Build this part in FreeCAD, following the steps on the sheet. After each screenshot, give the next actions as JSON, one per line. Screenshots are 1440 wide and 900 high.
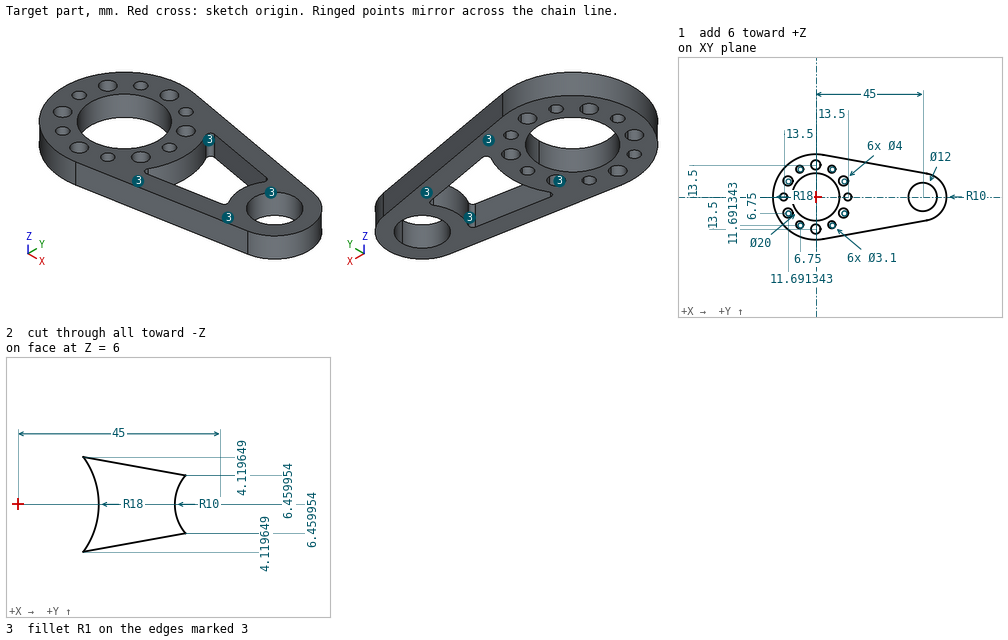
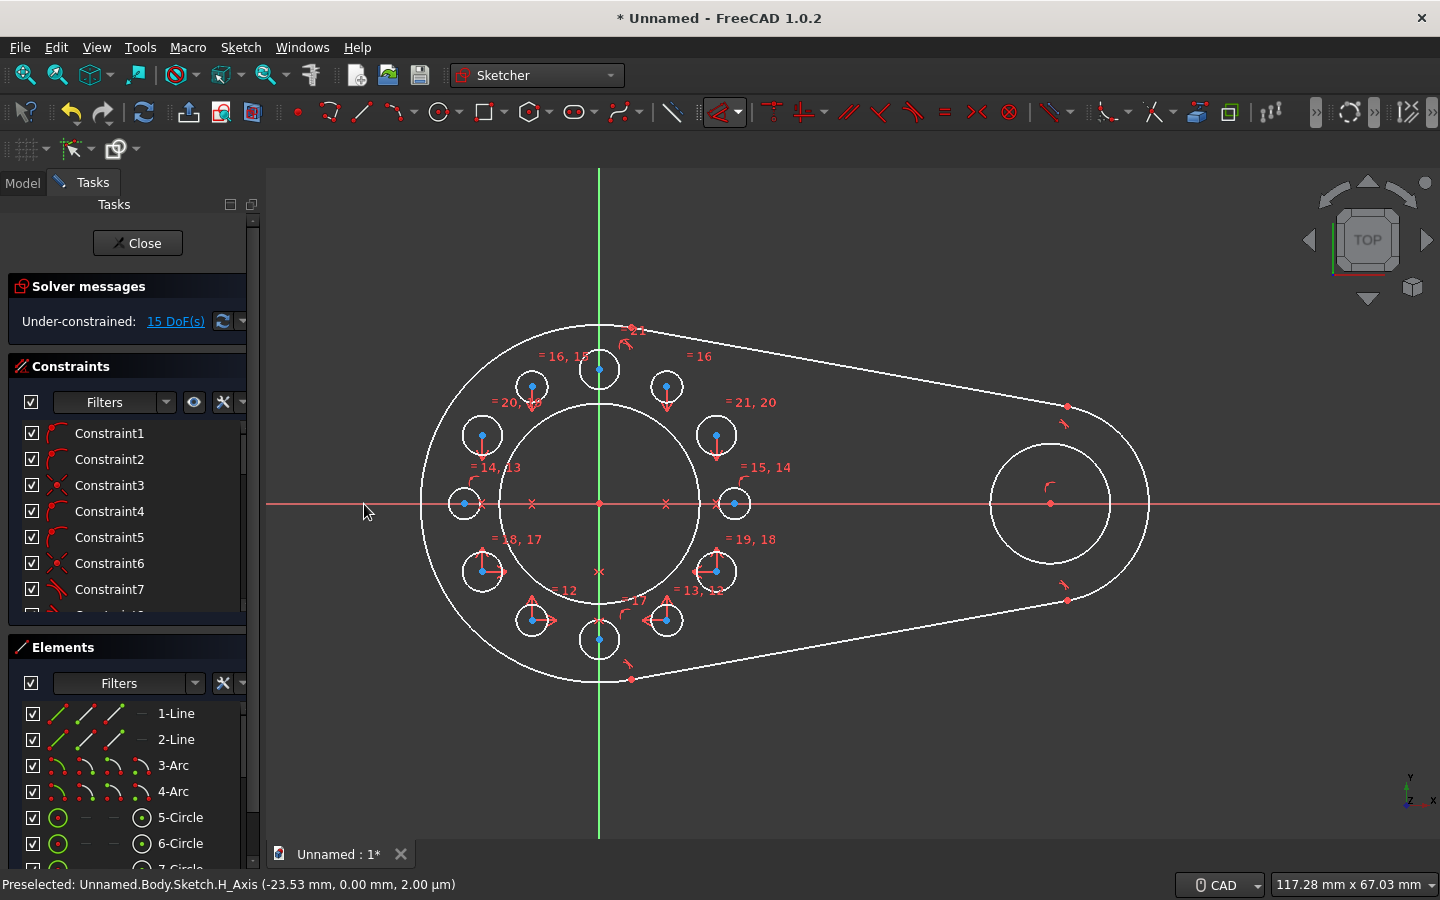
{"action": "left_click", "coordinate": [463, 388]}
{"action": "left_click", "coordinate": [439, 367]}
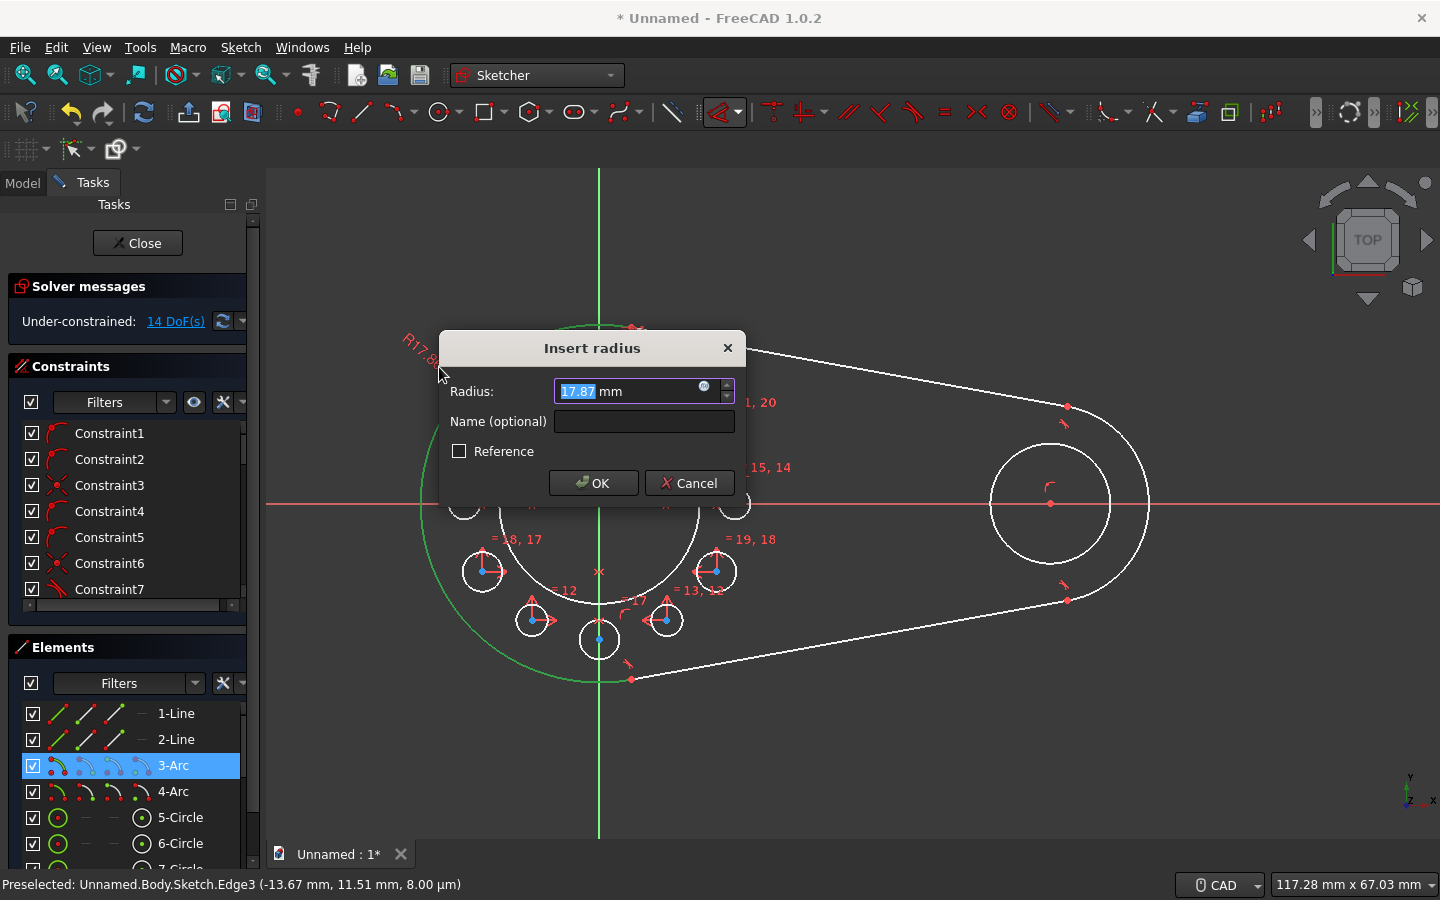
{"action": "type", "text": "18"}
{"action": "key", "text": "Return"}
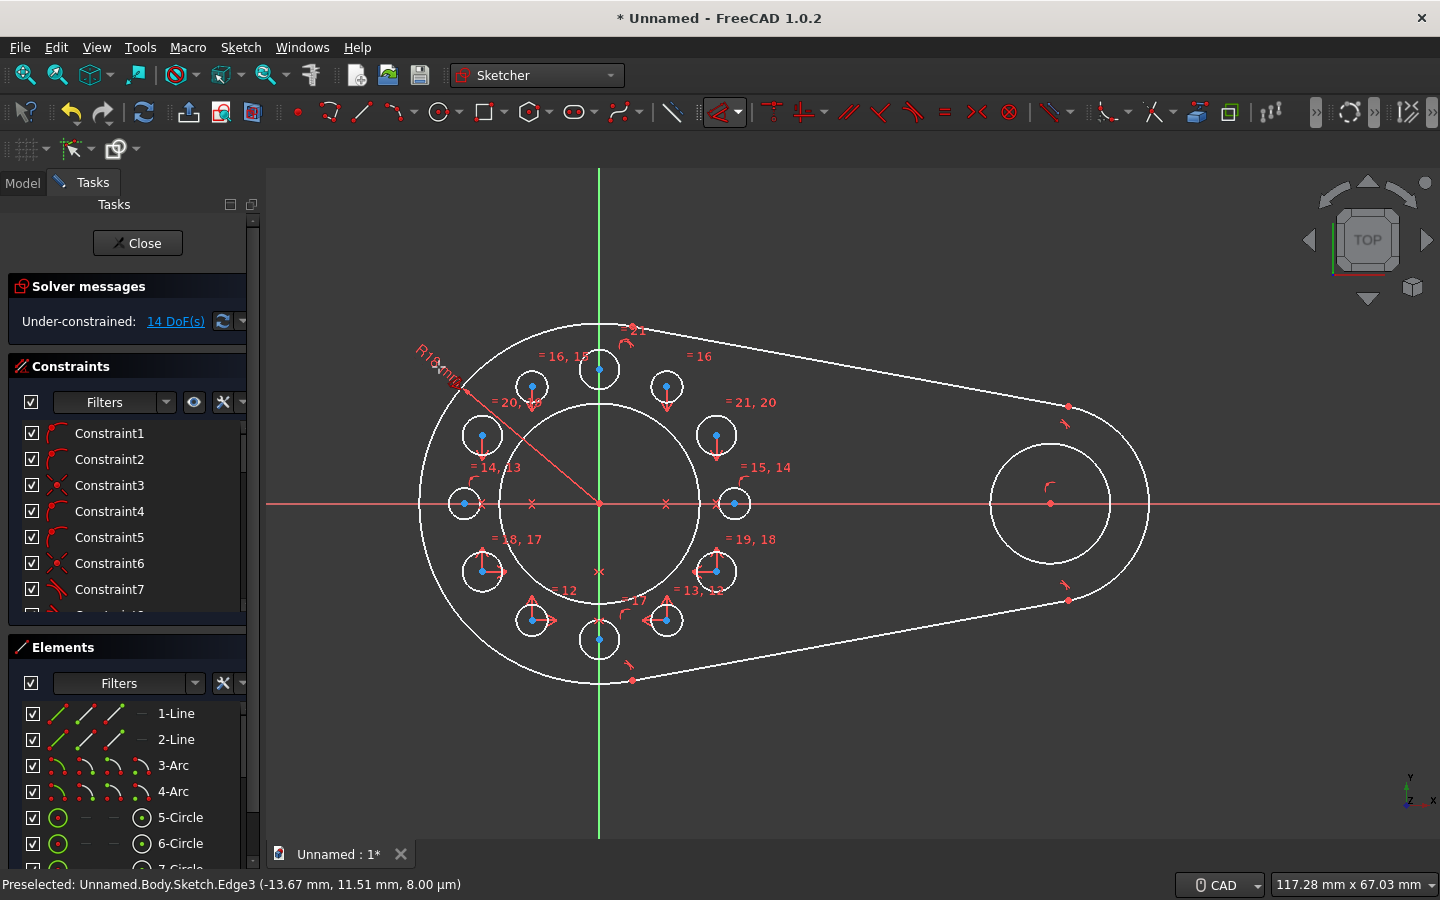
{"action": "left_click", "coordinate": [1134, 556]}
{"action": "left_click", "coordinate": [1161, 573]}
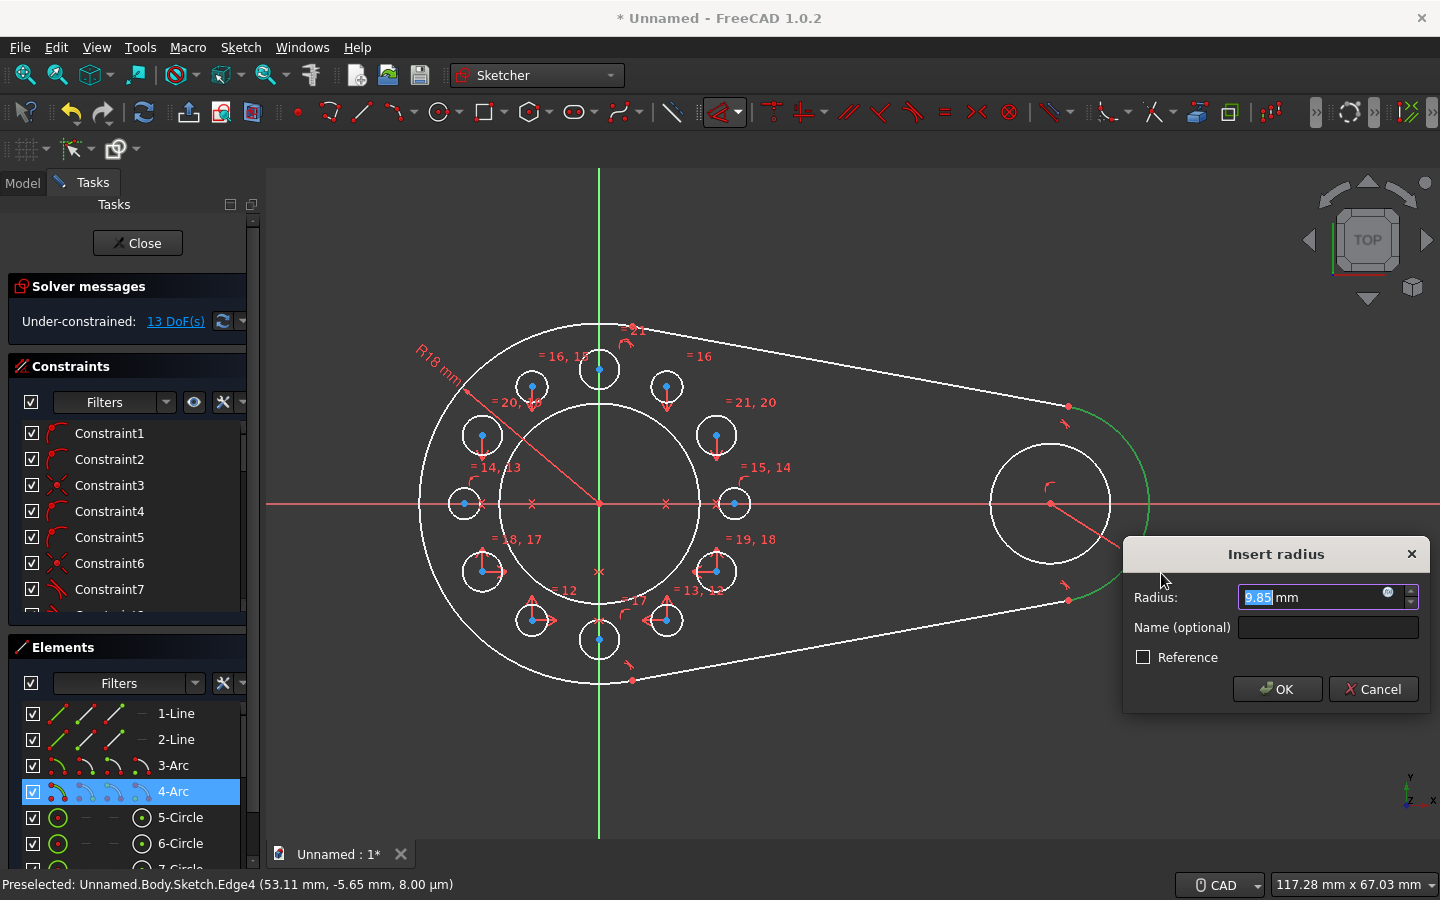
{"action": "type", "text": "10"}
{"action": "key", "text": "Return"}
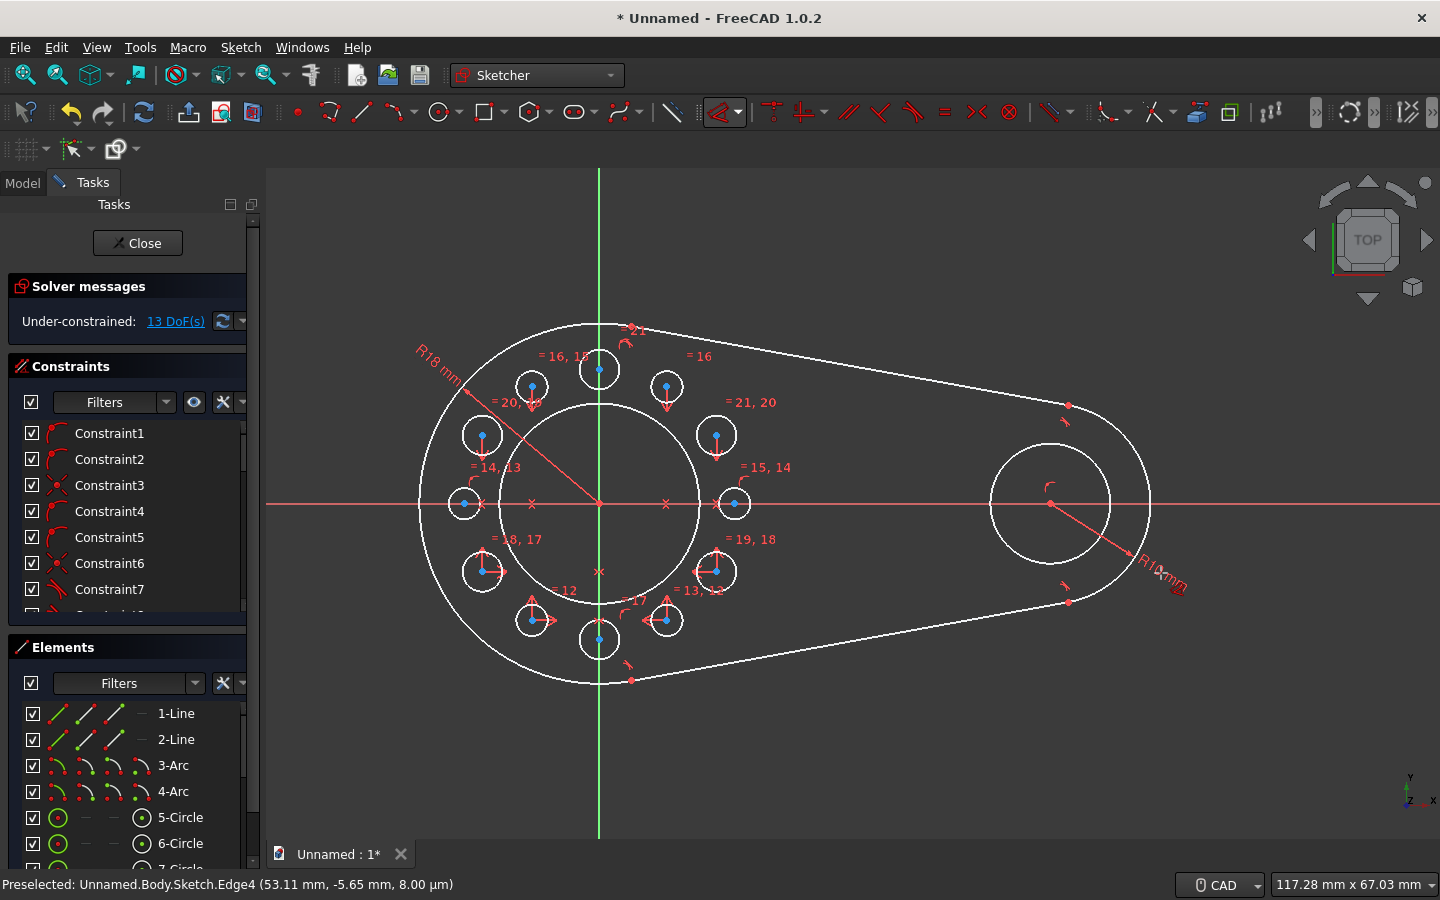
{"action": "scroll", "coordinate": [543, 609], "scroll_direction": "up", "scroll_amount": 2}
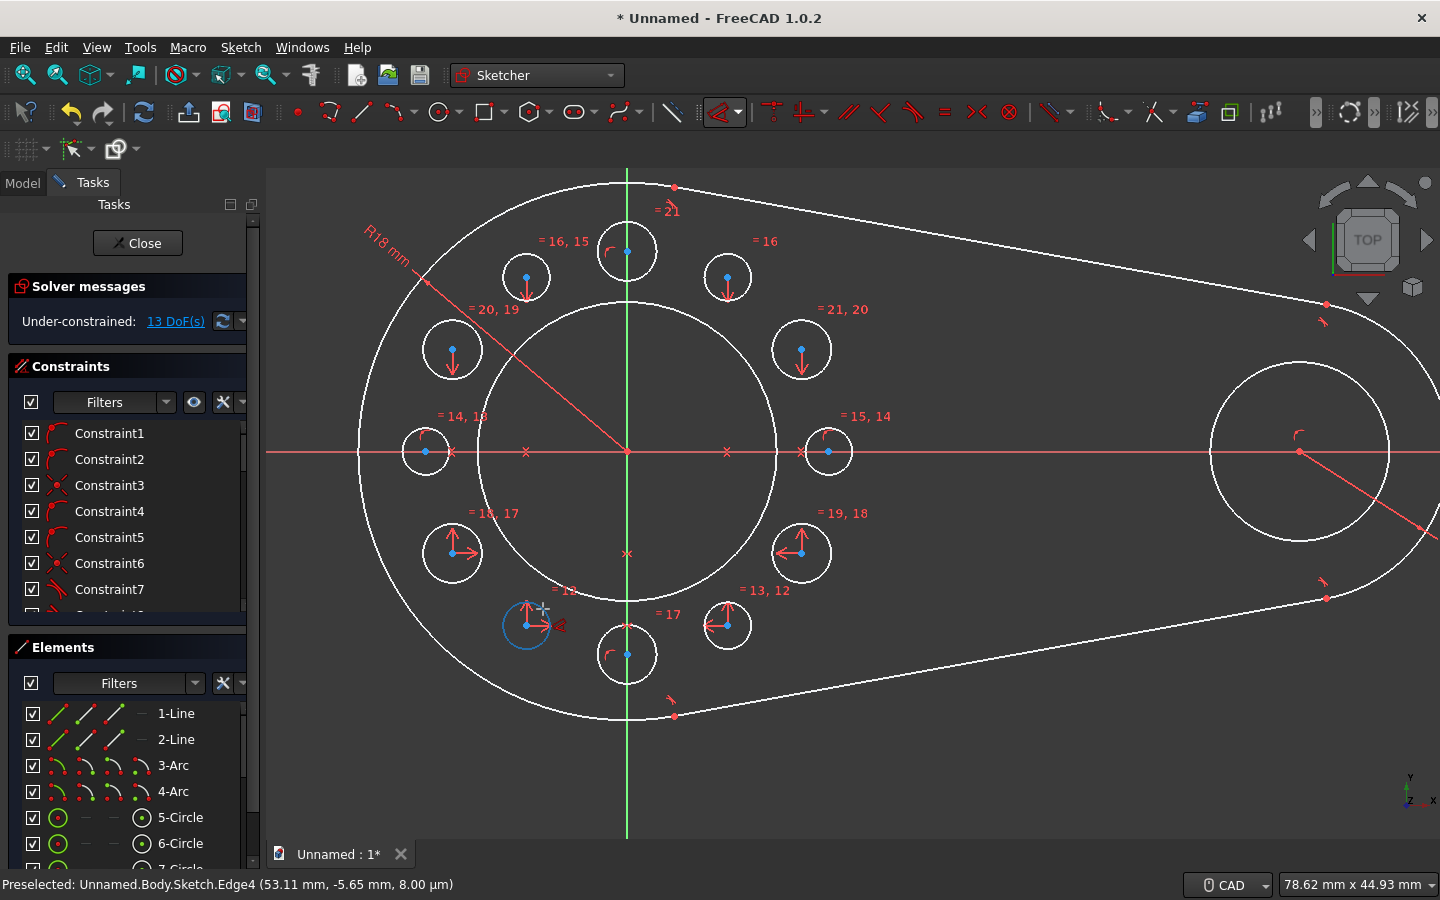
{"action": "left_click", "coordinate": [543, 609]}
{"action": "left_click", "coordinate": [580, 610]}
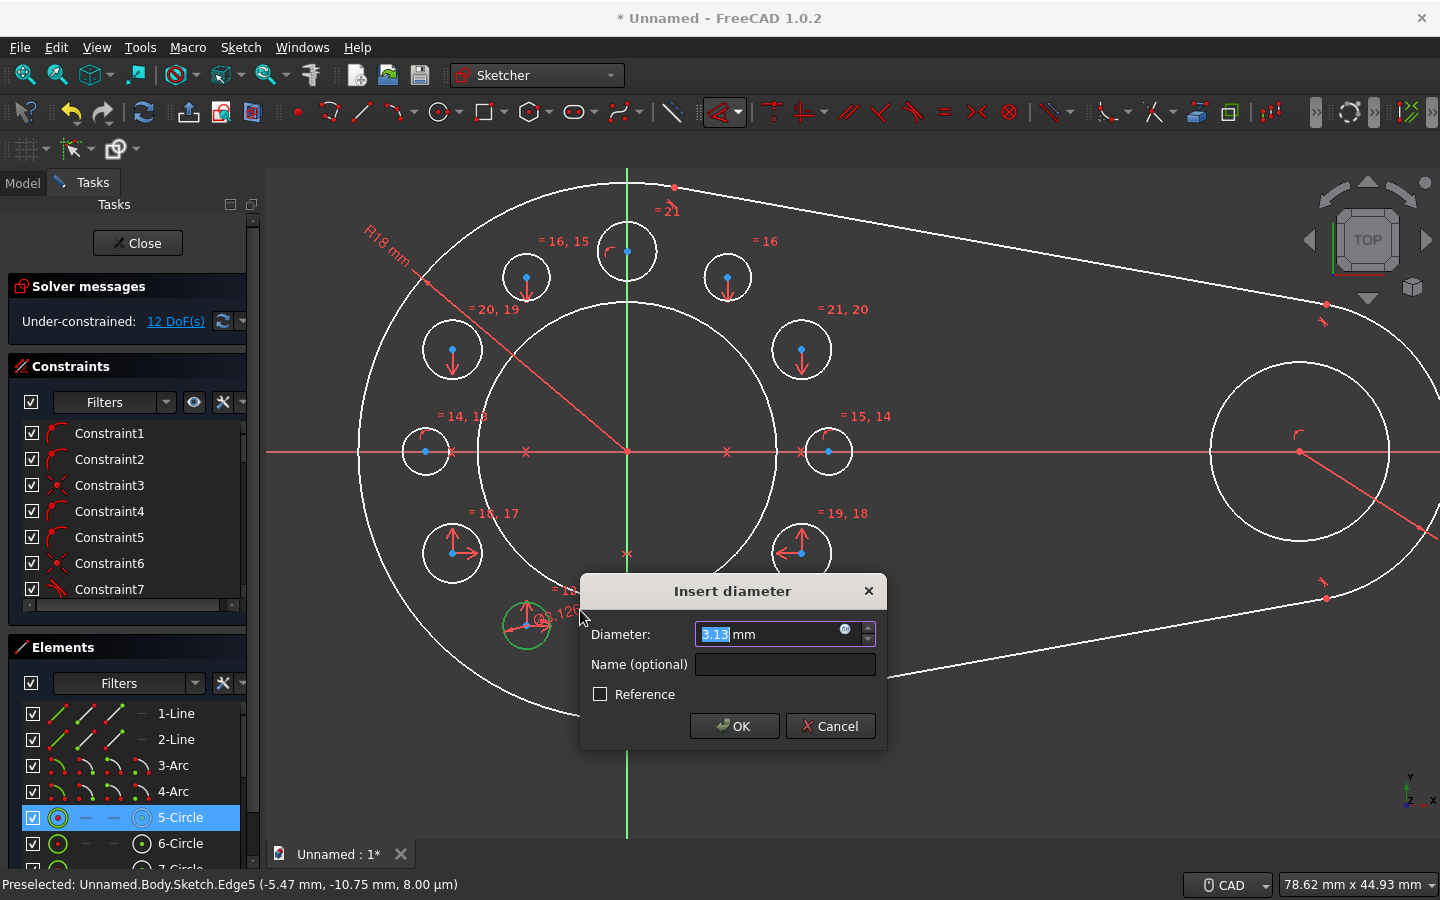
{"action": "type", "text": "3.1"}
{"action": "key", "text": "Return"}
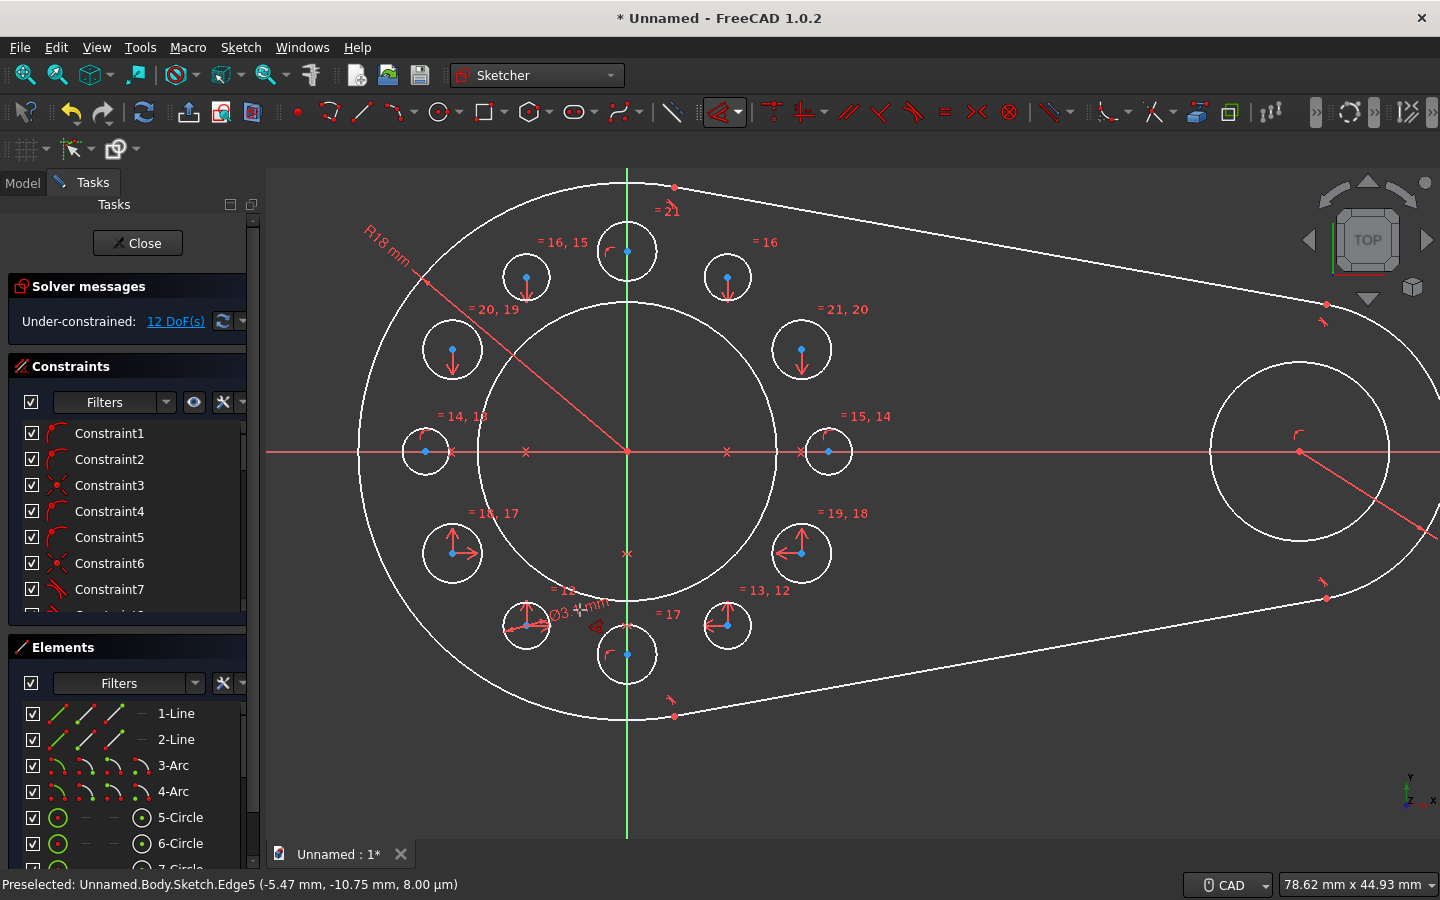
{"action": "left_click", "coordinate": [648, 634]}
{"action": "left_click", "coordinate": [671, 612]}